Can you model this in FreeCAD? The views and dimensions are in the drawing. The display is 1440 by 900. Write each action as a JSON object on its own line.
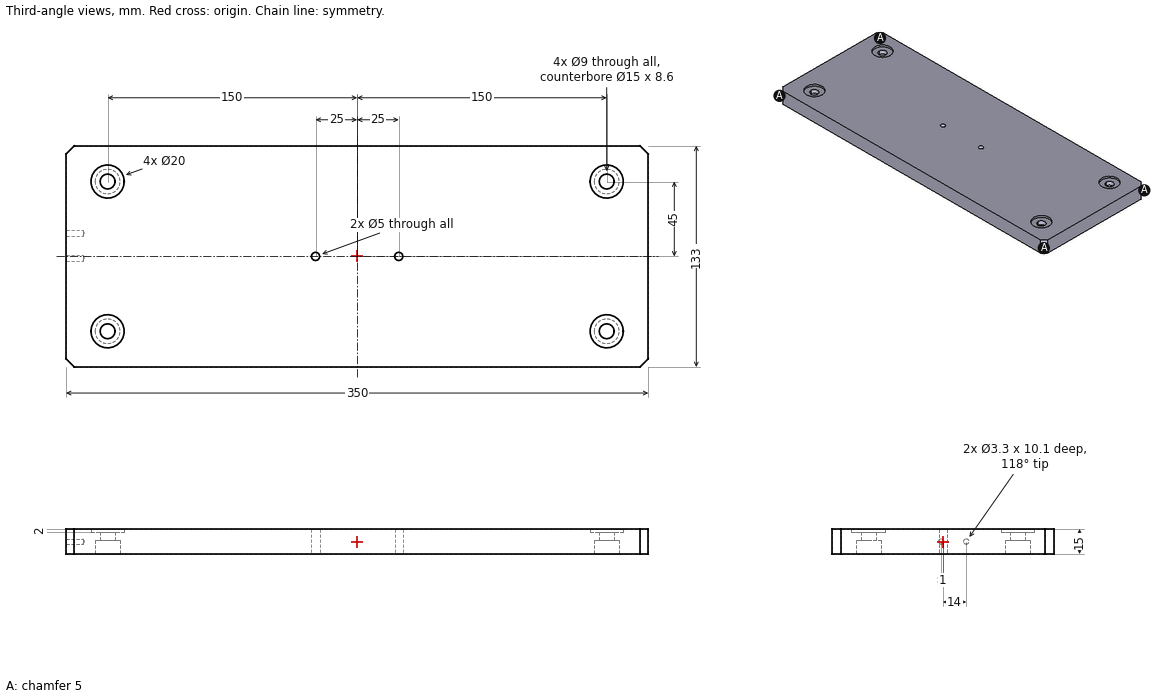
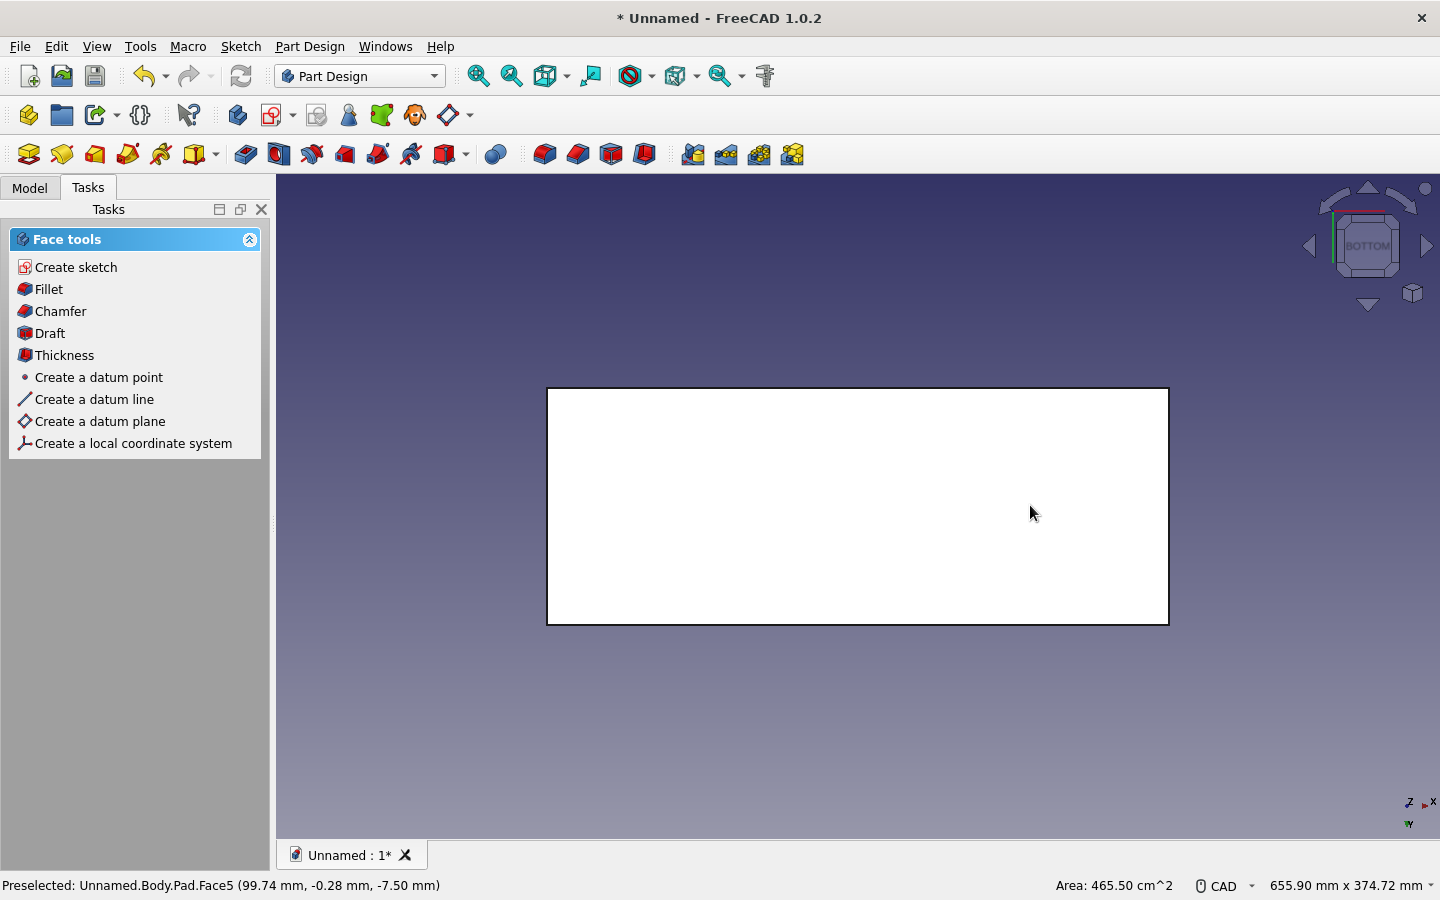
{"action": "left_click", "coordinate": [270, 116]}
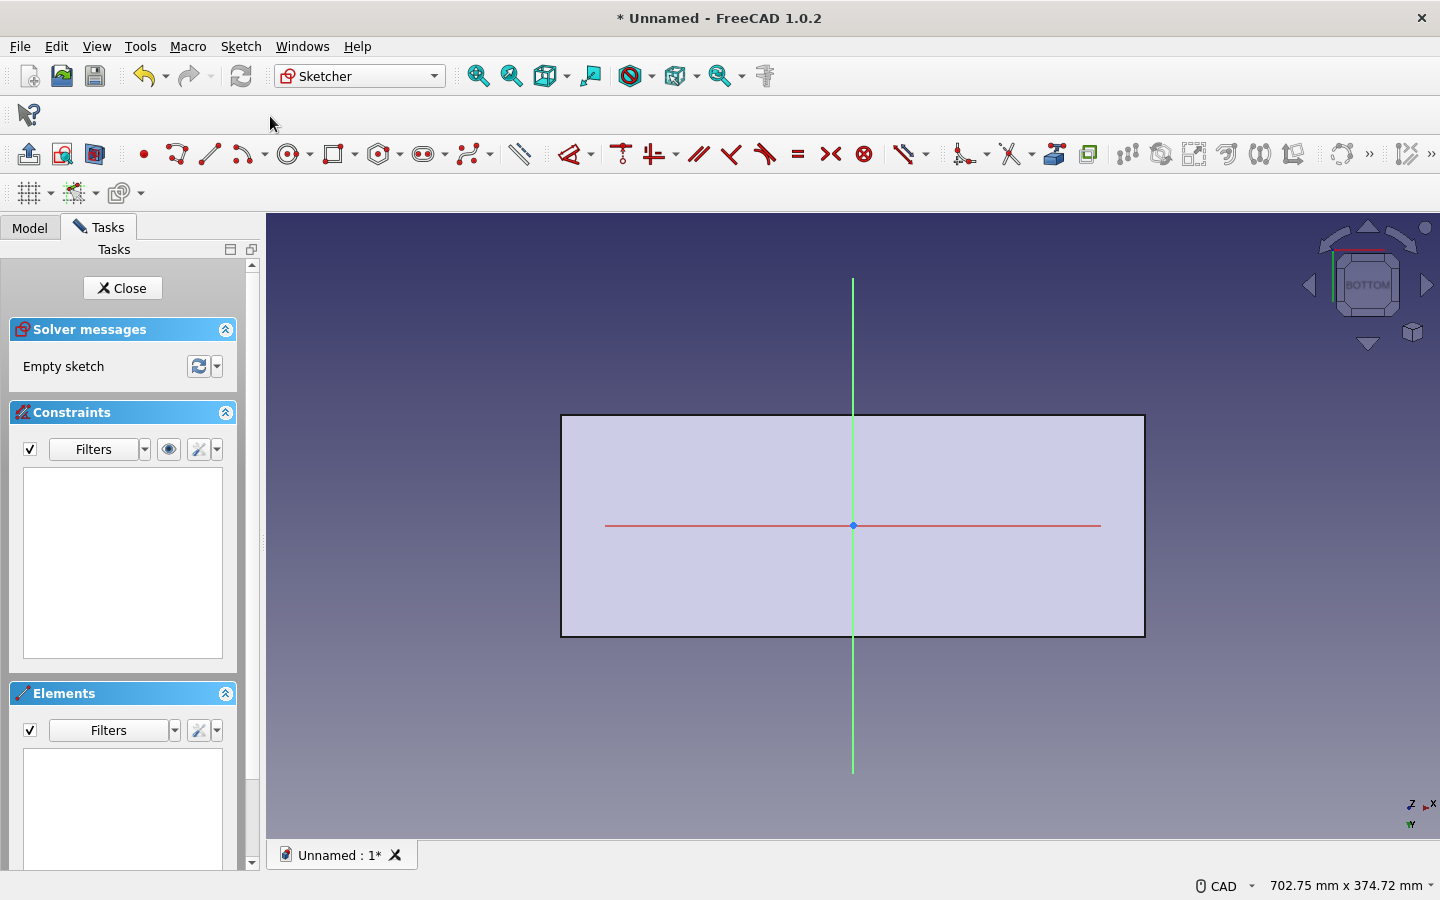
{"action": "left_click", "coordinate": [288, 154]}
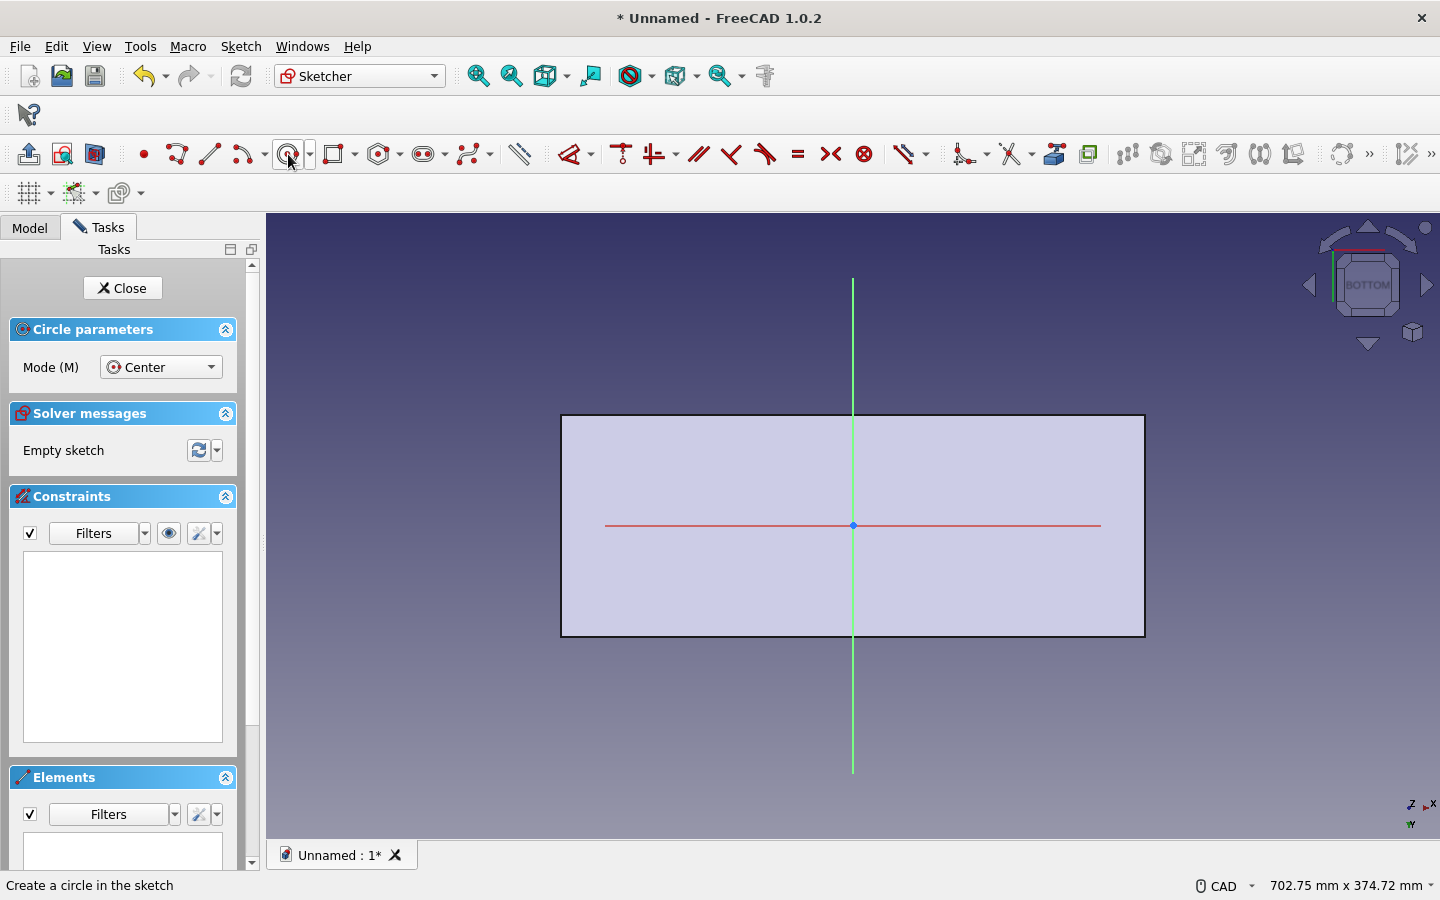
{"action": "scroll", "coordinate": [1104, 601], "scroll_direction": "up", "scroll_amount": 6}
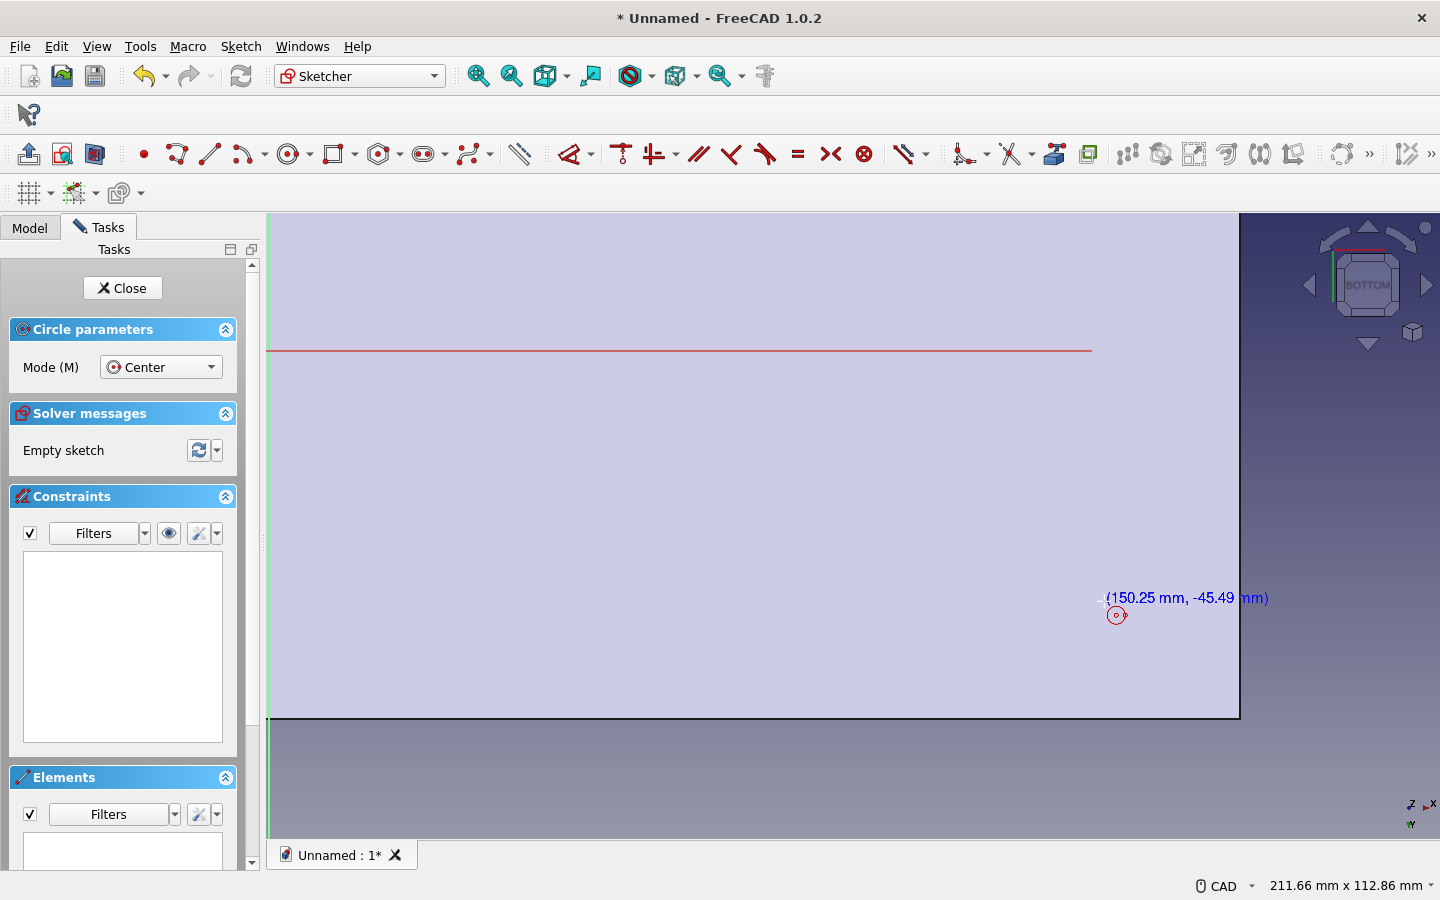
{"action": "left_click", "coordinate": [1101, 600]}
{"action": "mouse_move", "coordinate": [1119, 582]}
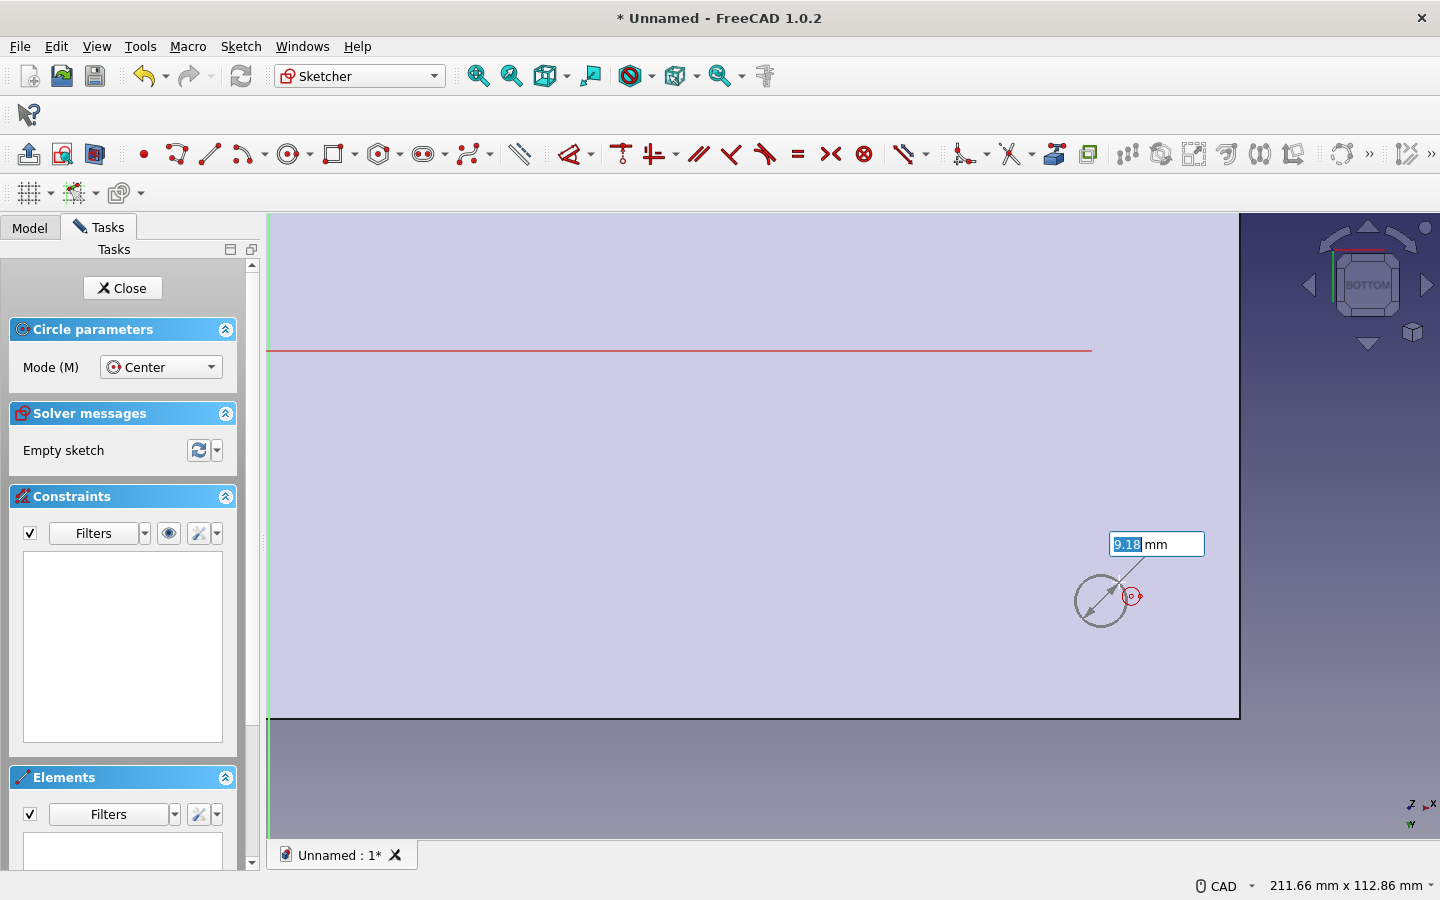
{"action": "type", "text": "9"}
{"action": "key", "text": "Return"}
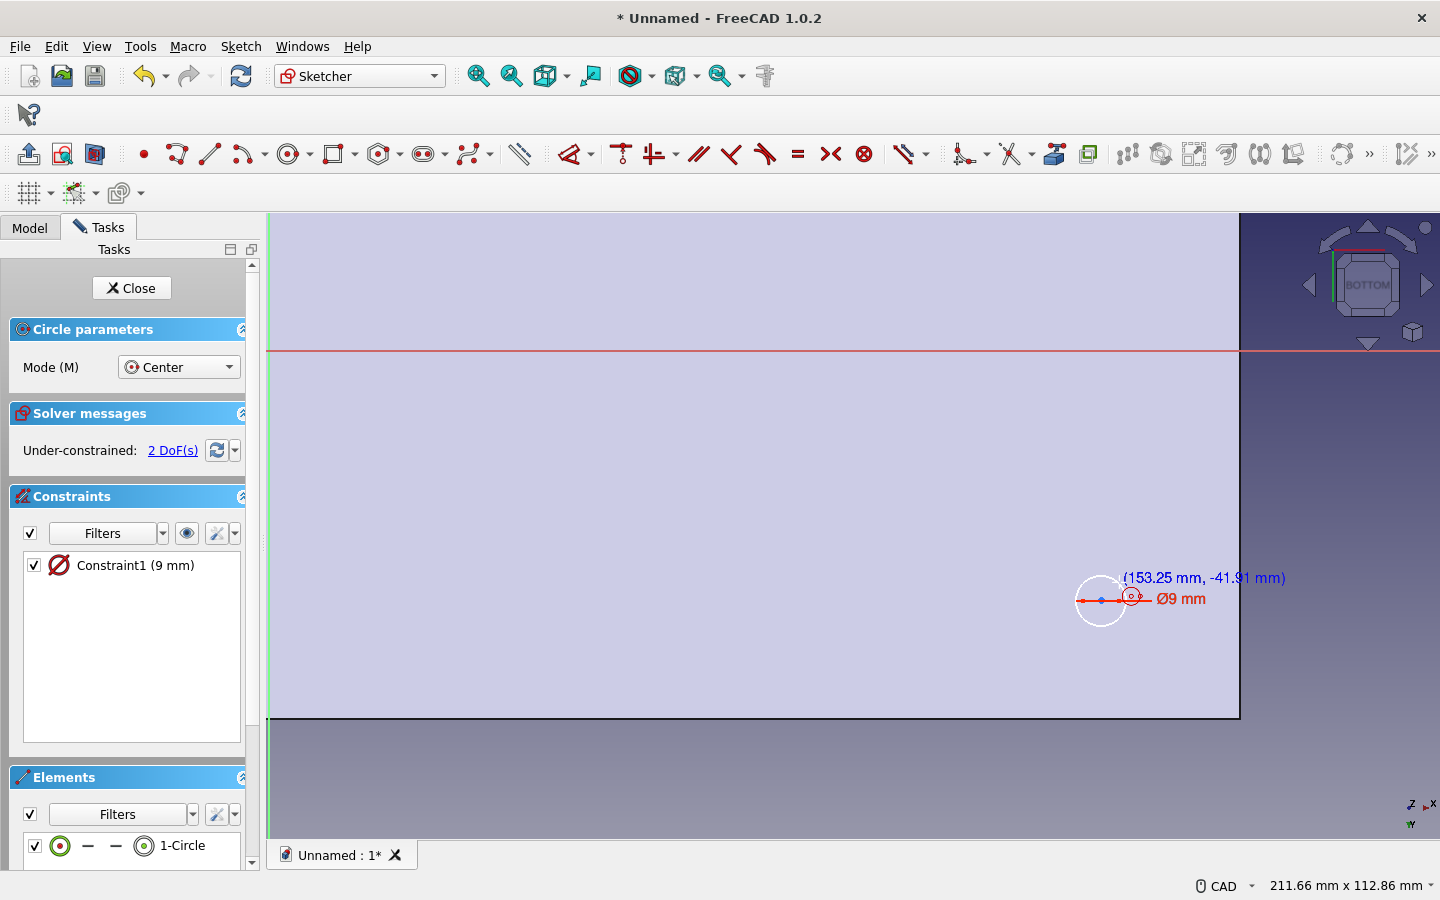
{"action": "scroll", "coordinate": [1085, 628], "scroll_direction": "down", "scroll_amount": 5}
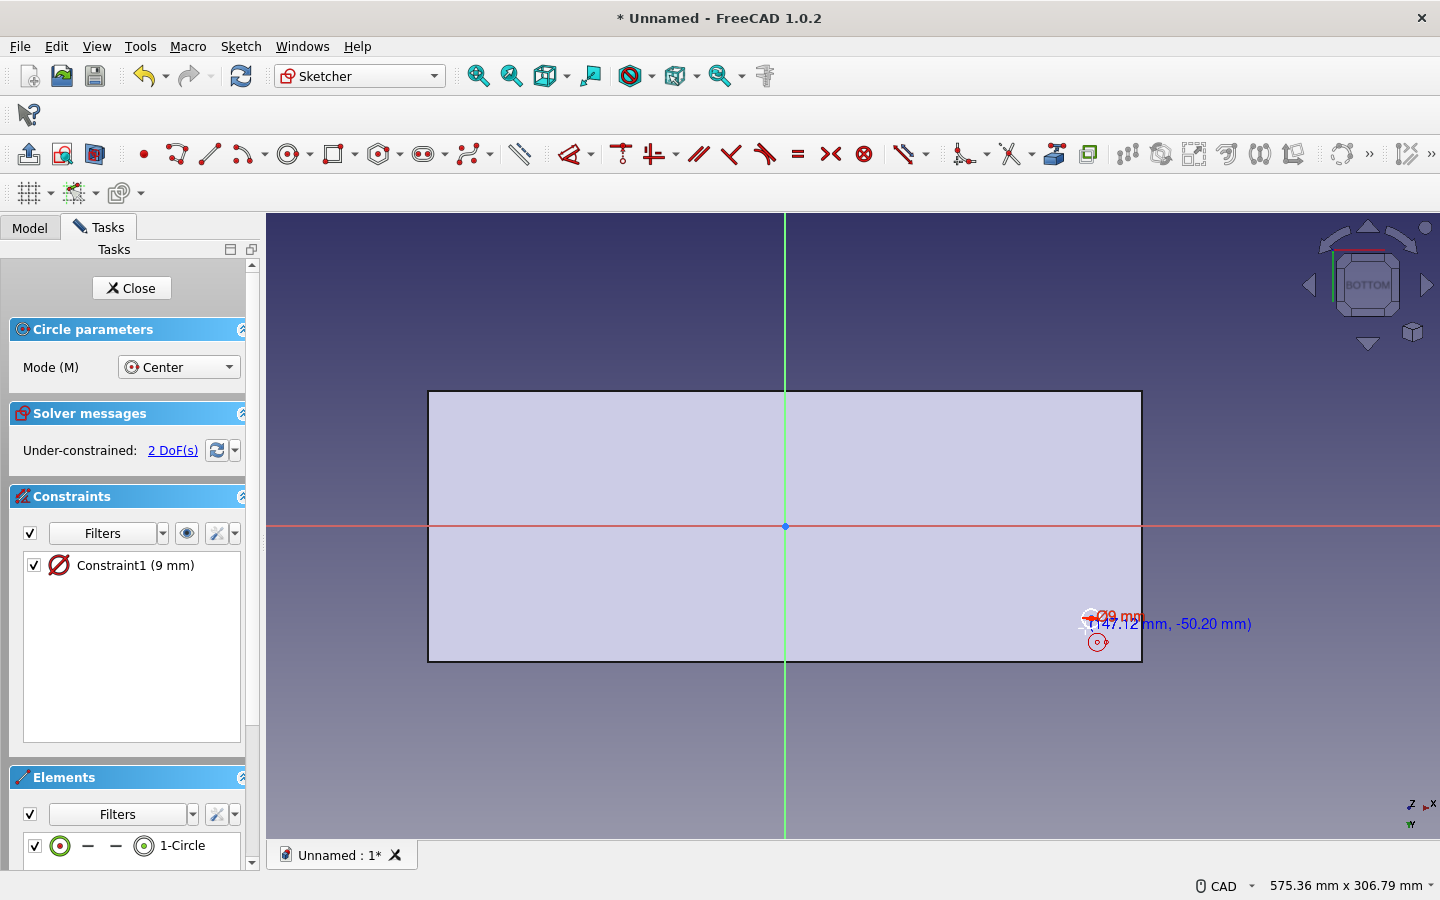
{"action": "scroll", "coordinate": [1091, 435], "scroll_direction": "up", "scroll_amount": 5}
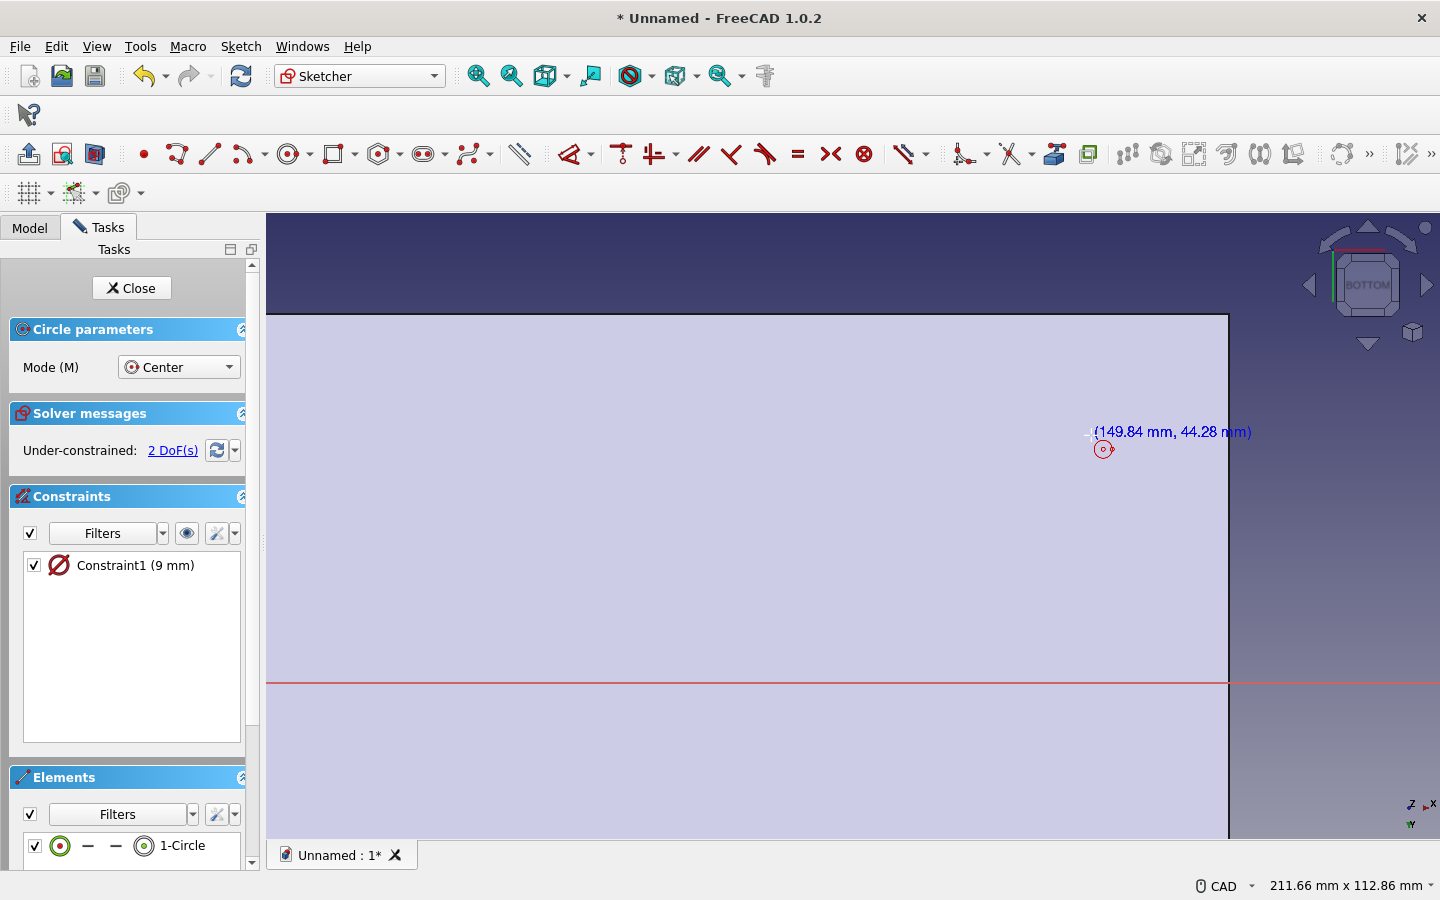
{"action": "left_click", "coordinate": [1091, 433]}
{"action": "mouse_move", "coordinate": [1108, 415]}